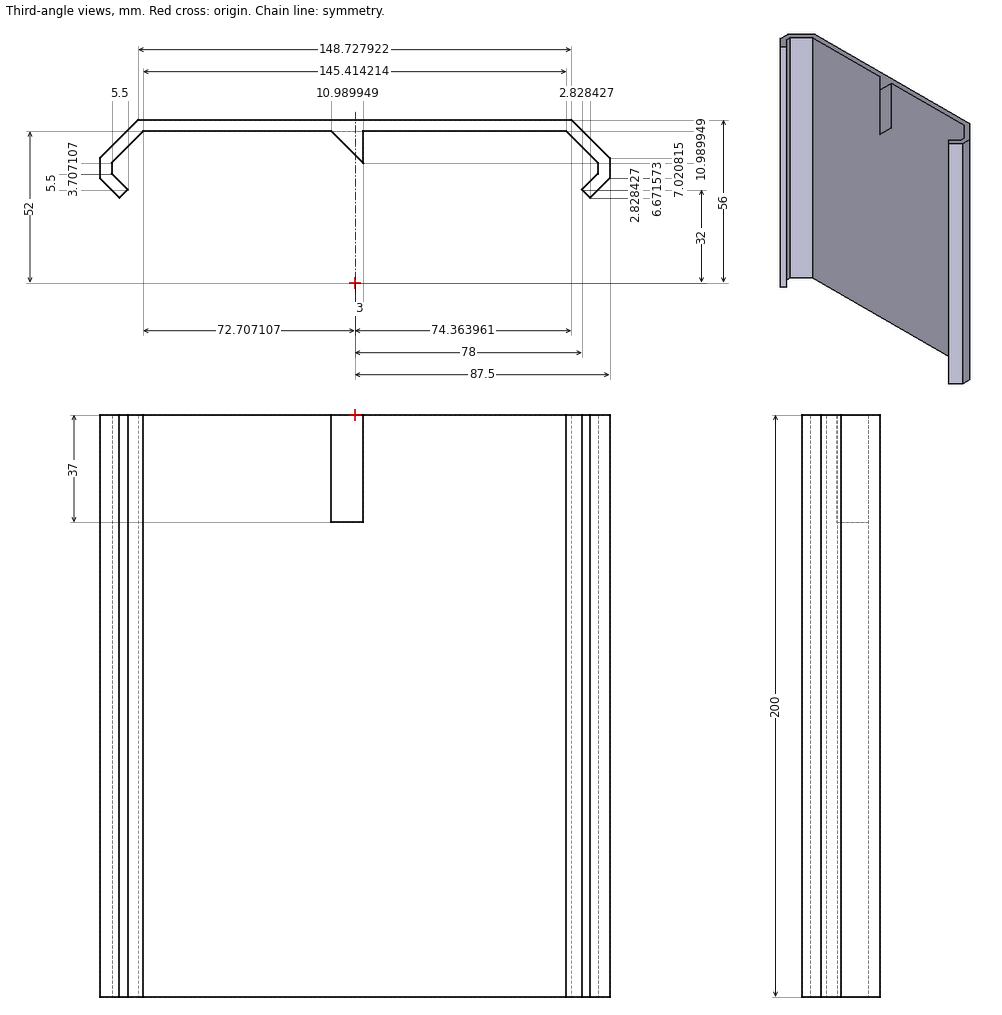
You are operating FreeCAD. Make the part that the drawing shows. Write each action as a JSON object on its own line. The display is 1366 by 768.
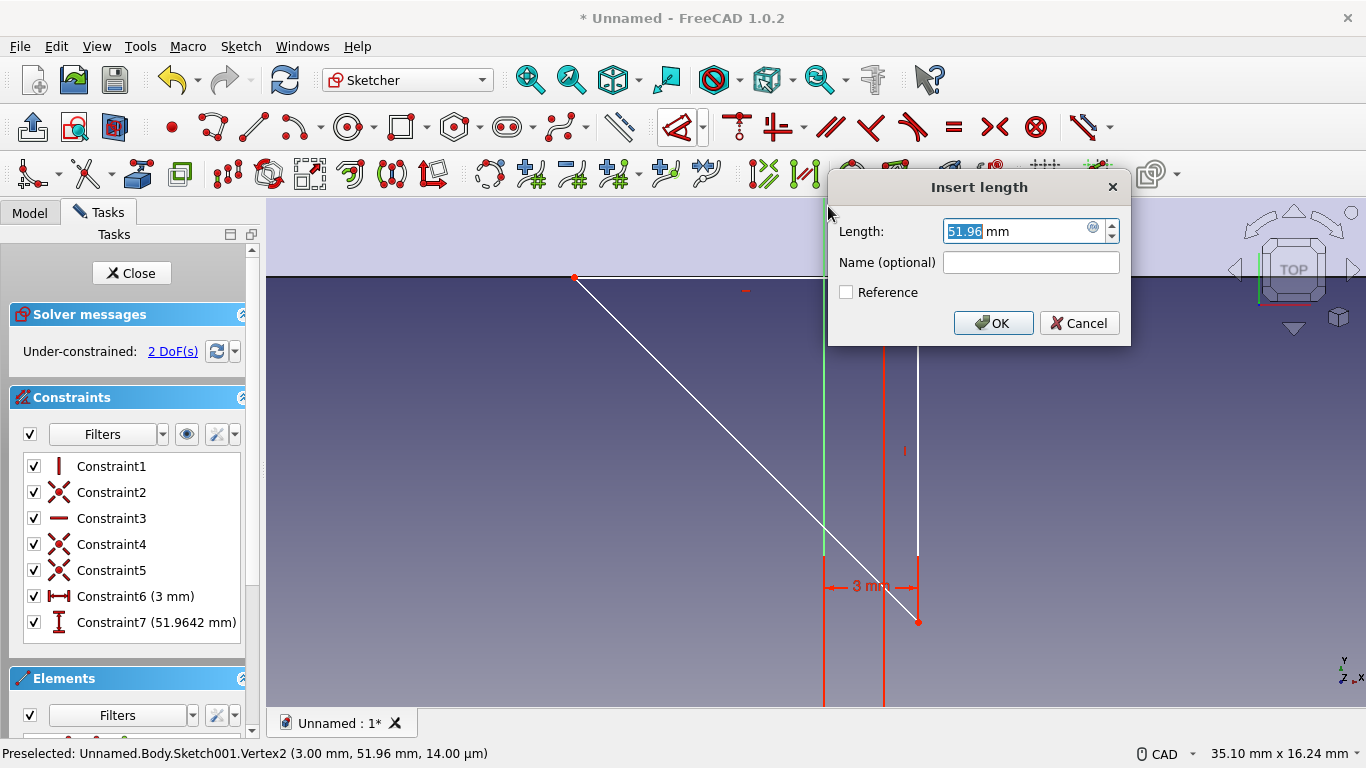
{"action": "type", "text": "52"}
{"action": "key", "text": "Return"}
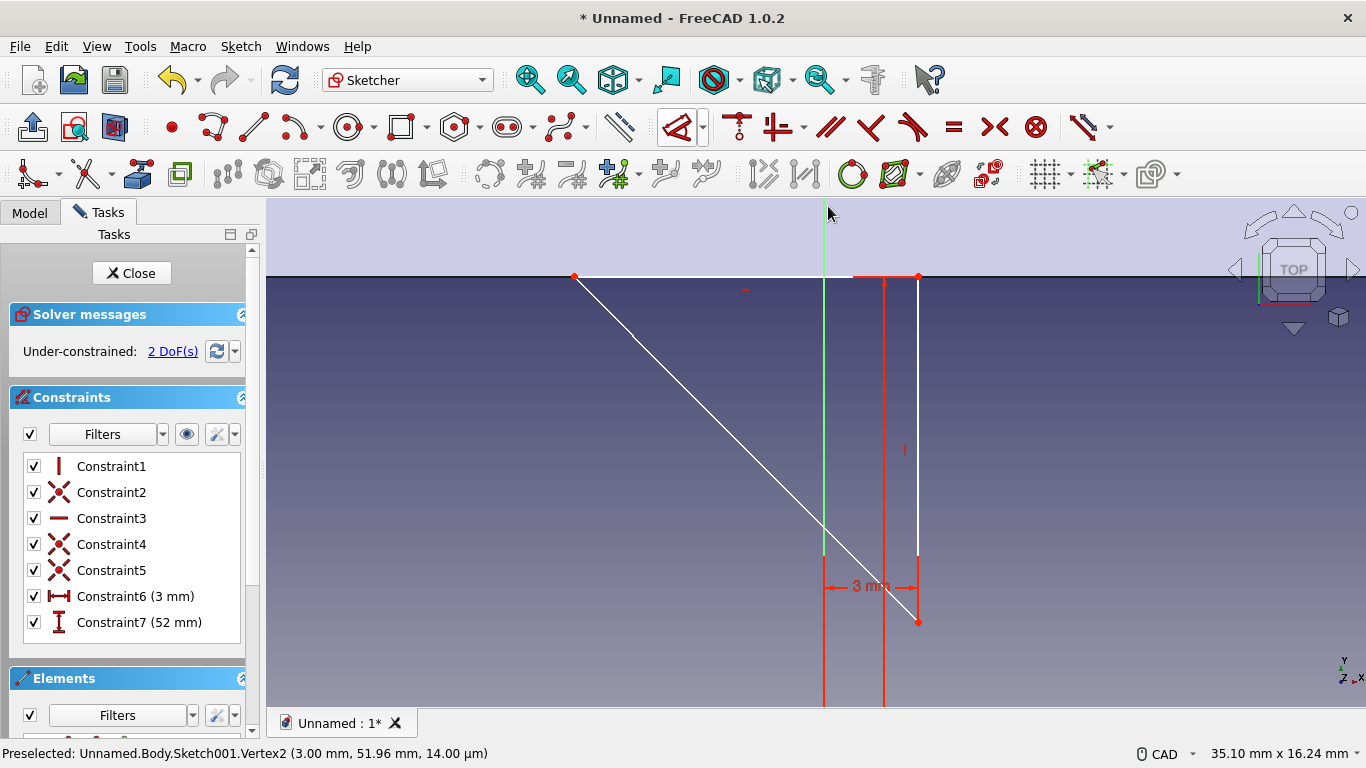
{"action": "left_click", "coordinate": [918, 518]}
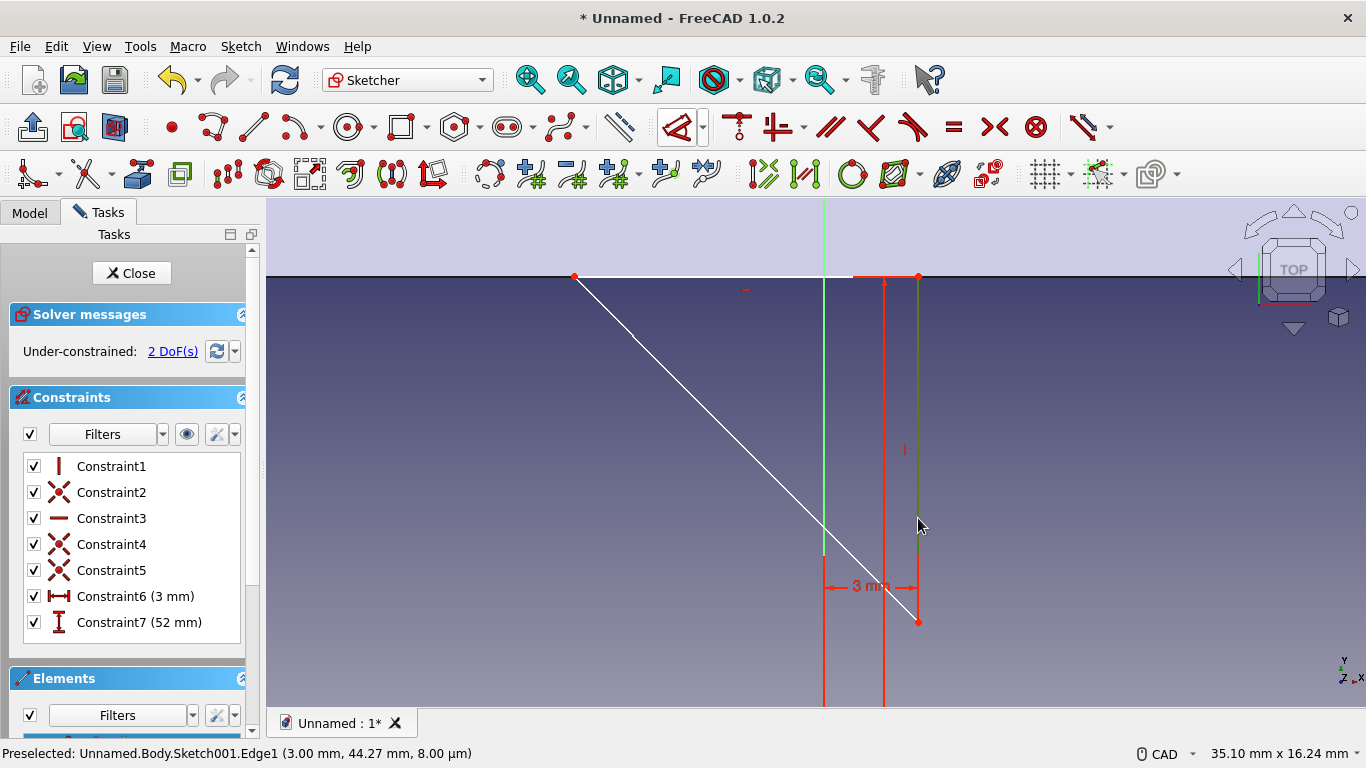
{"action": "key", "text": "i"}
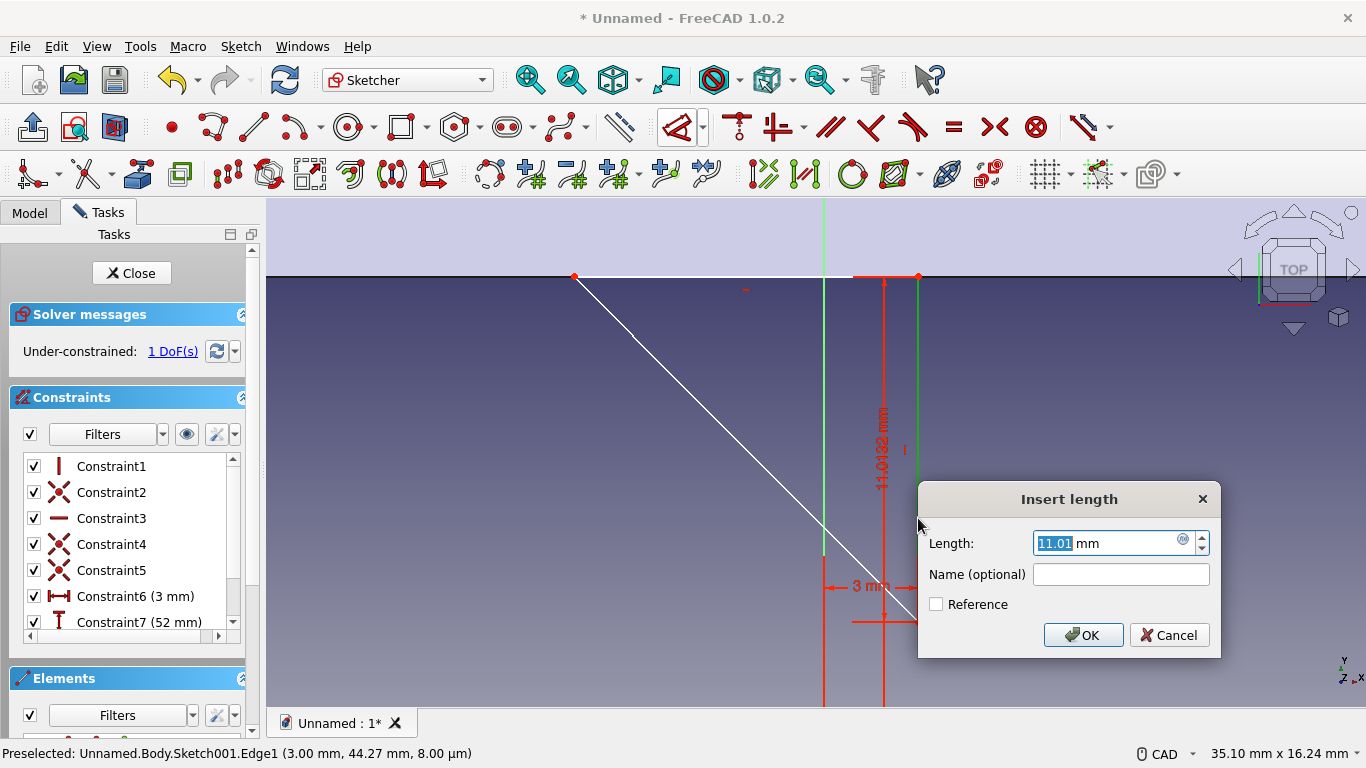
{"action": "type", "text": "10.989949"}
{"action": "key", "text": "Return"}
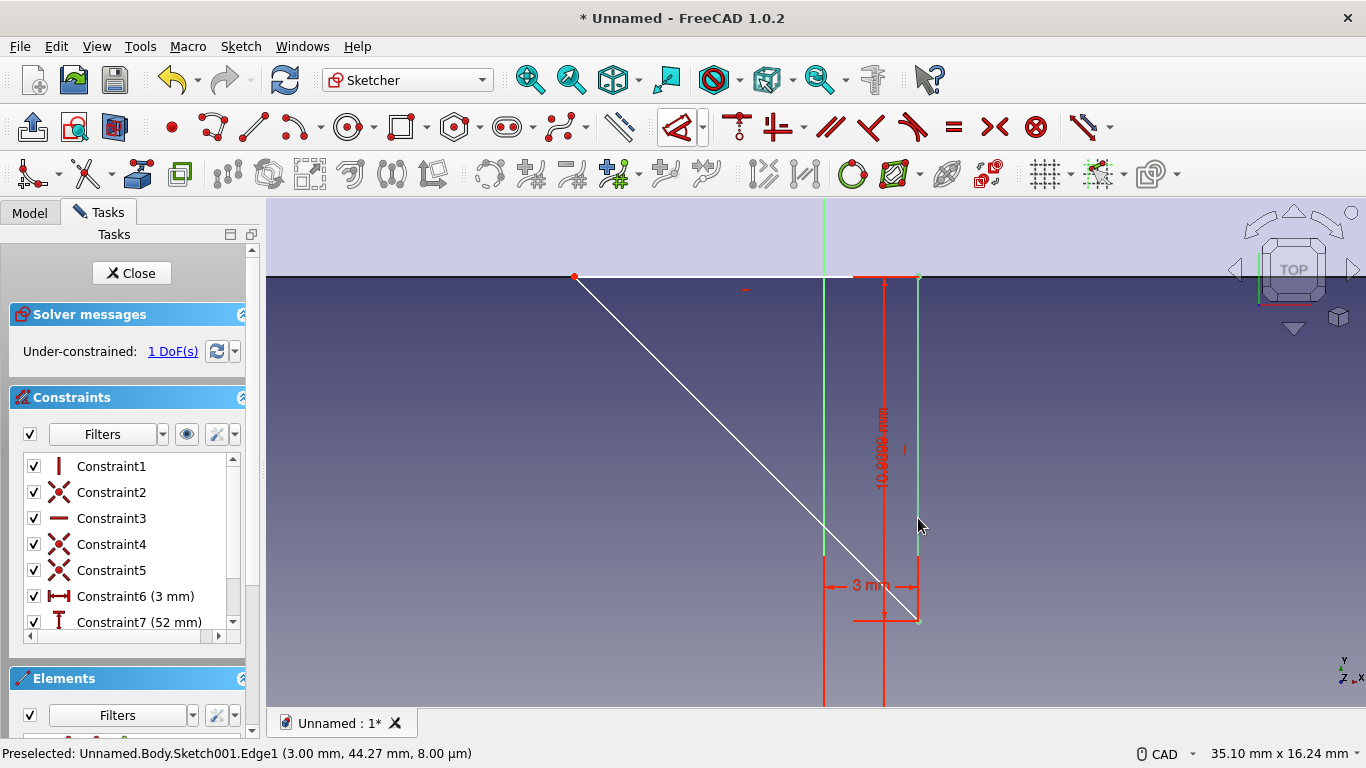
{"action": "scroll", "coordinate": [815, 277], "scroll_direction": "up", "scroll_amount": 2}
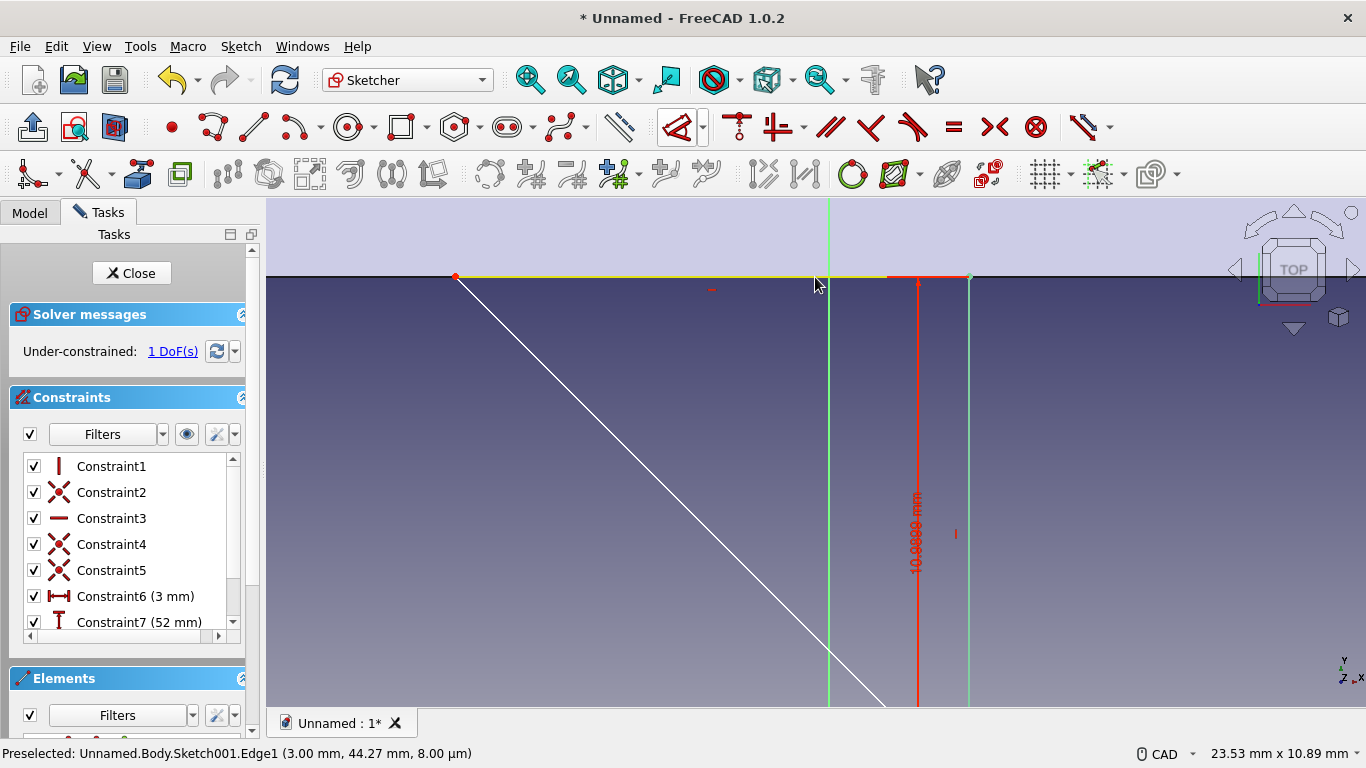
{"action": "left_click", "coordinate": [815, 277]}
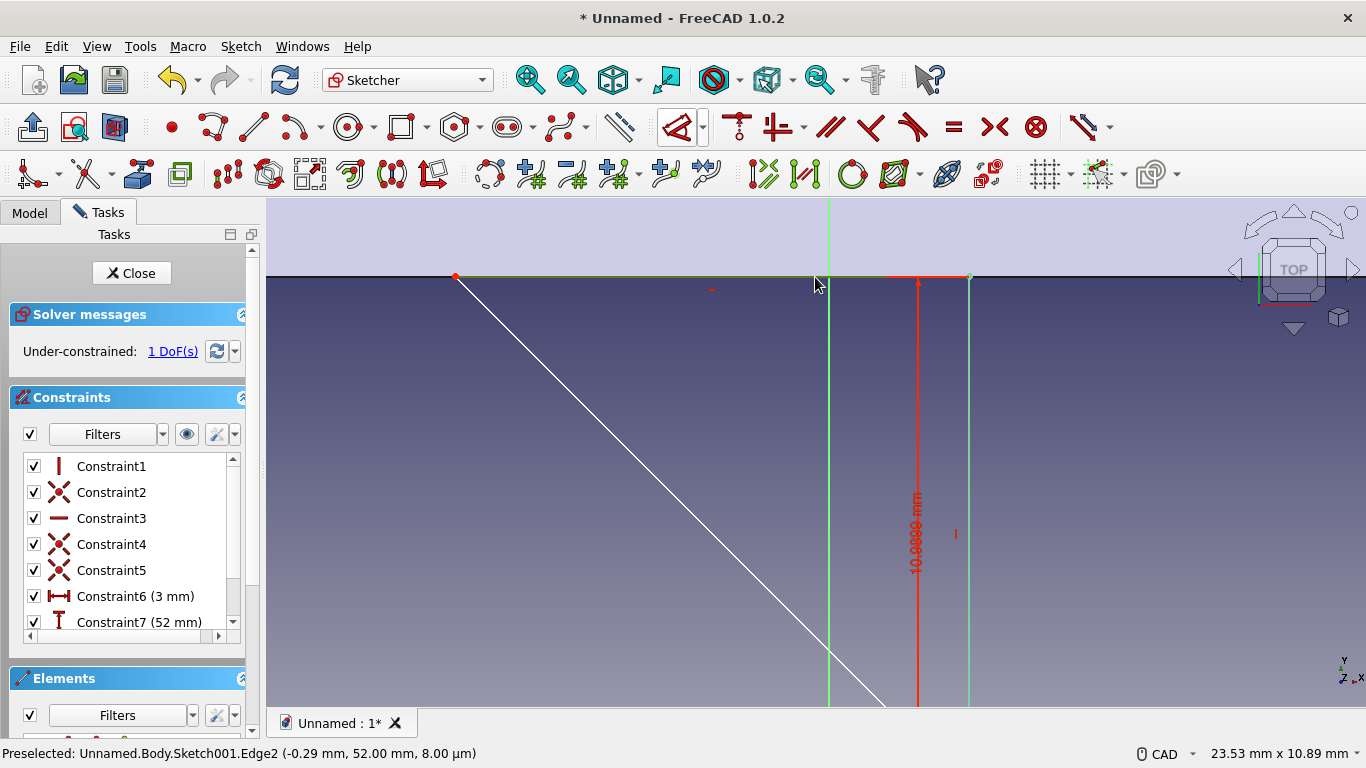
{"action": "left_click", "coordinate": [702, 128]}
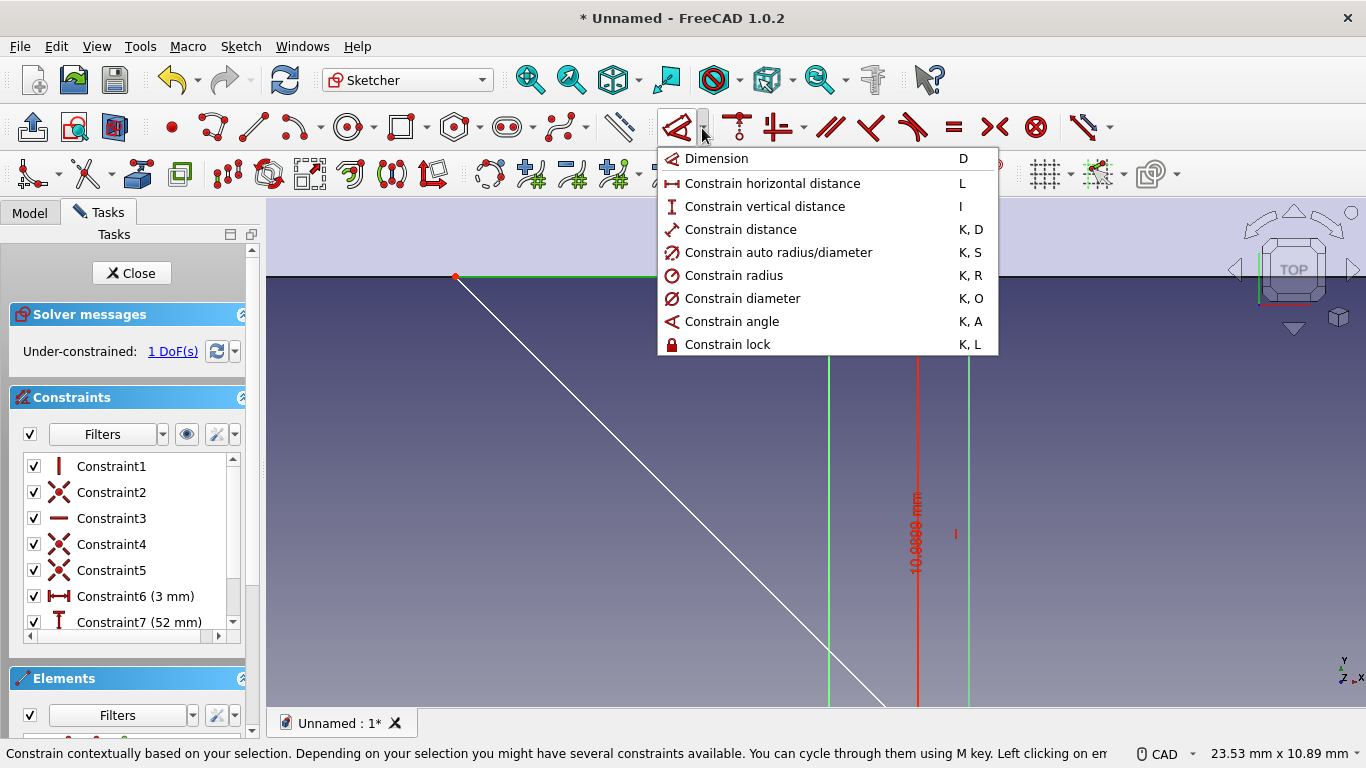
{"action": "left_click", "coordinate": [828, 184]}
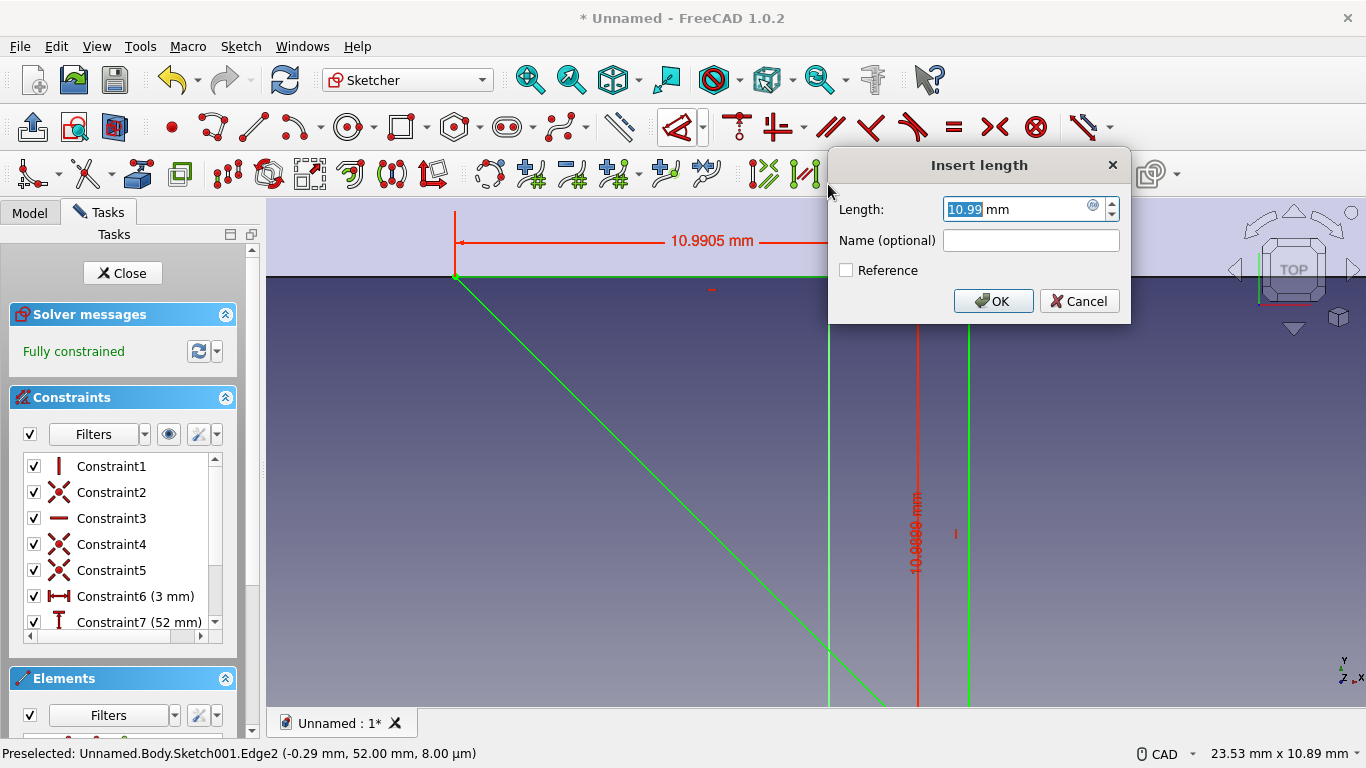
{"action": "type", "text": "10.989949"}
{"action": "key", "text": "Return"}